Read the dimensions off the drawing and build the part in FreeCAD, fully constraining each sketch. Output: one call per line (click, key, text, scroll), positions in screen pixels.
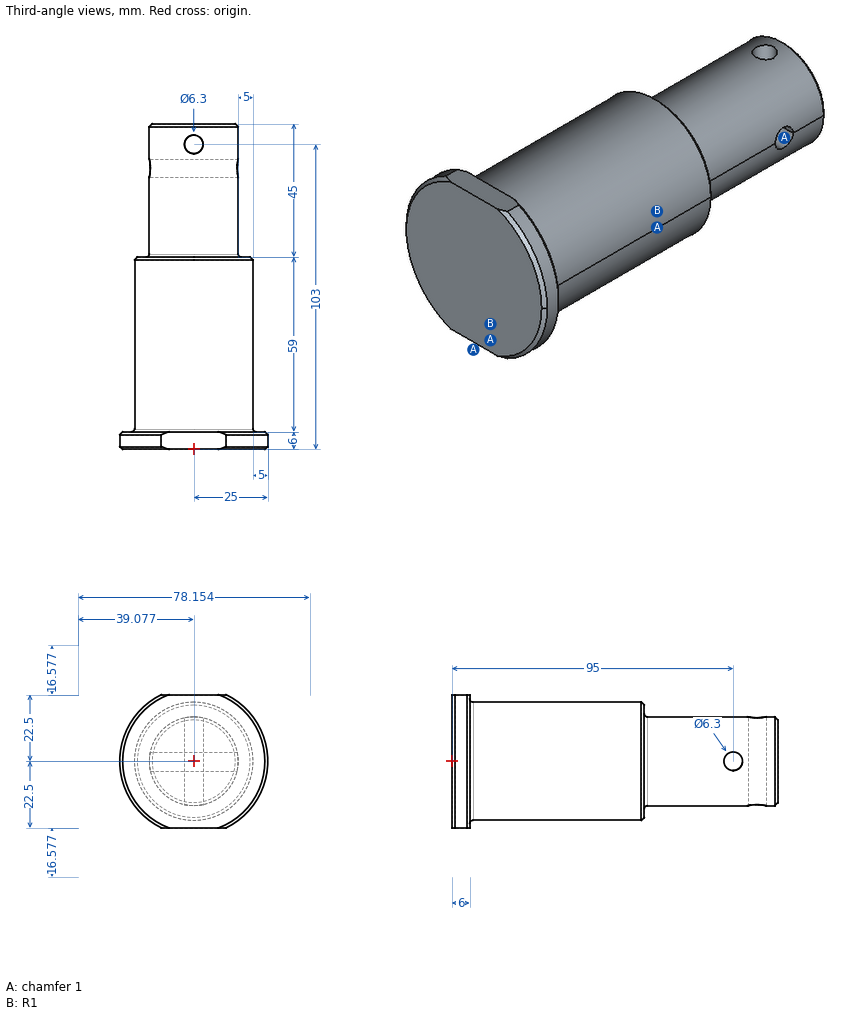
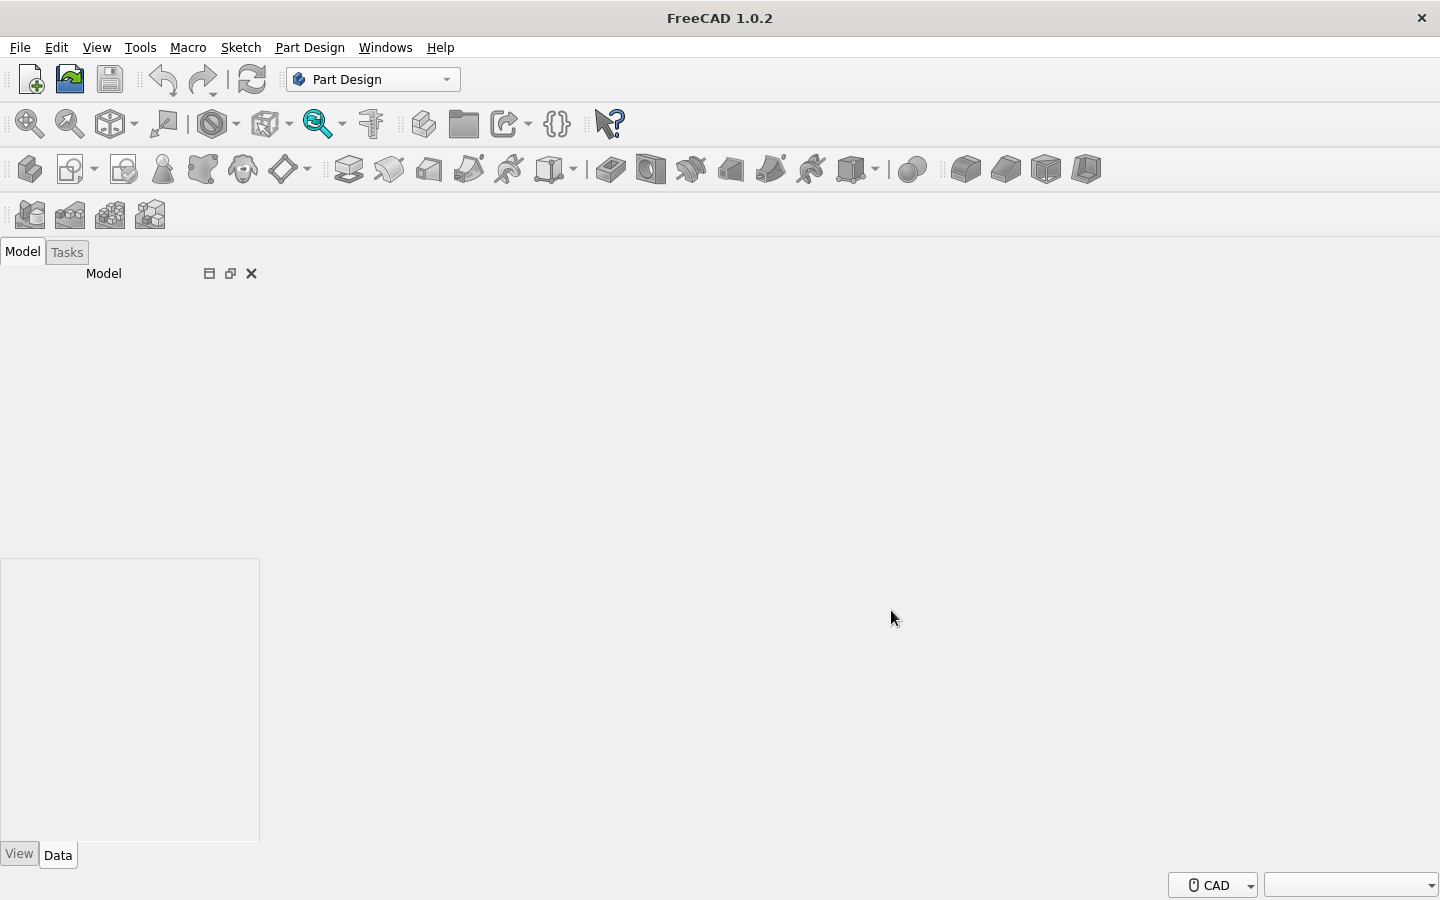
key(ctrl+n)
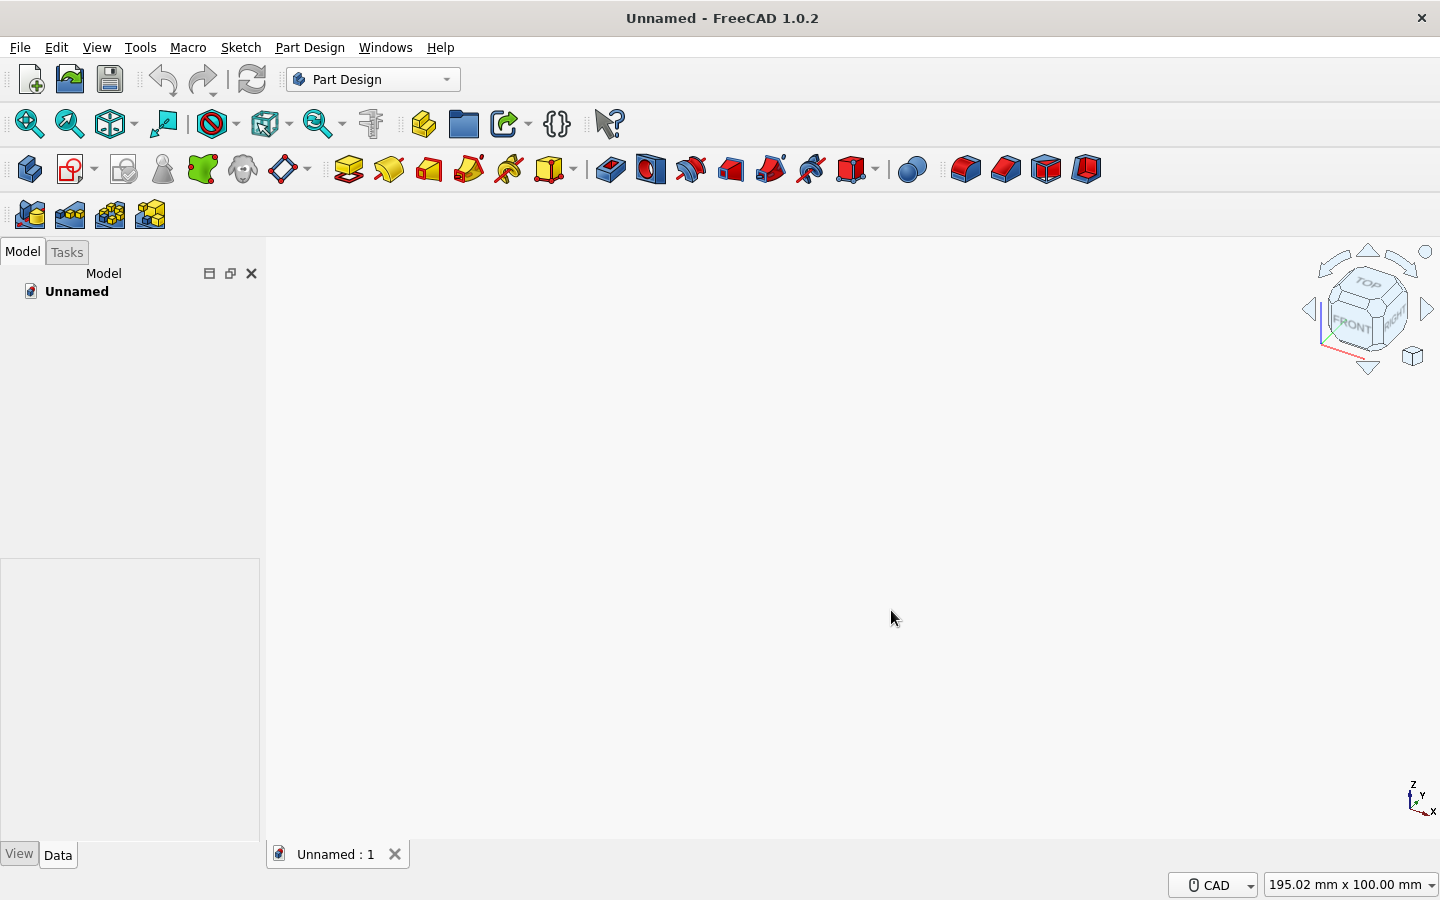
click(70, 170)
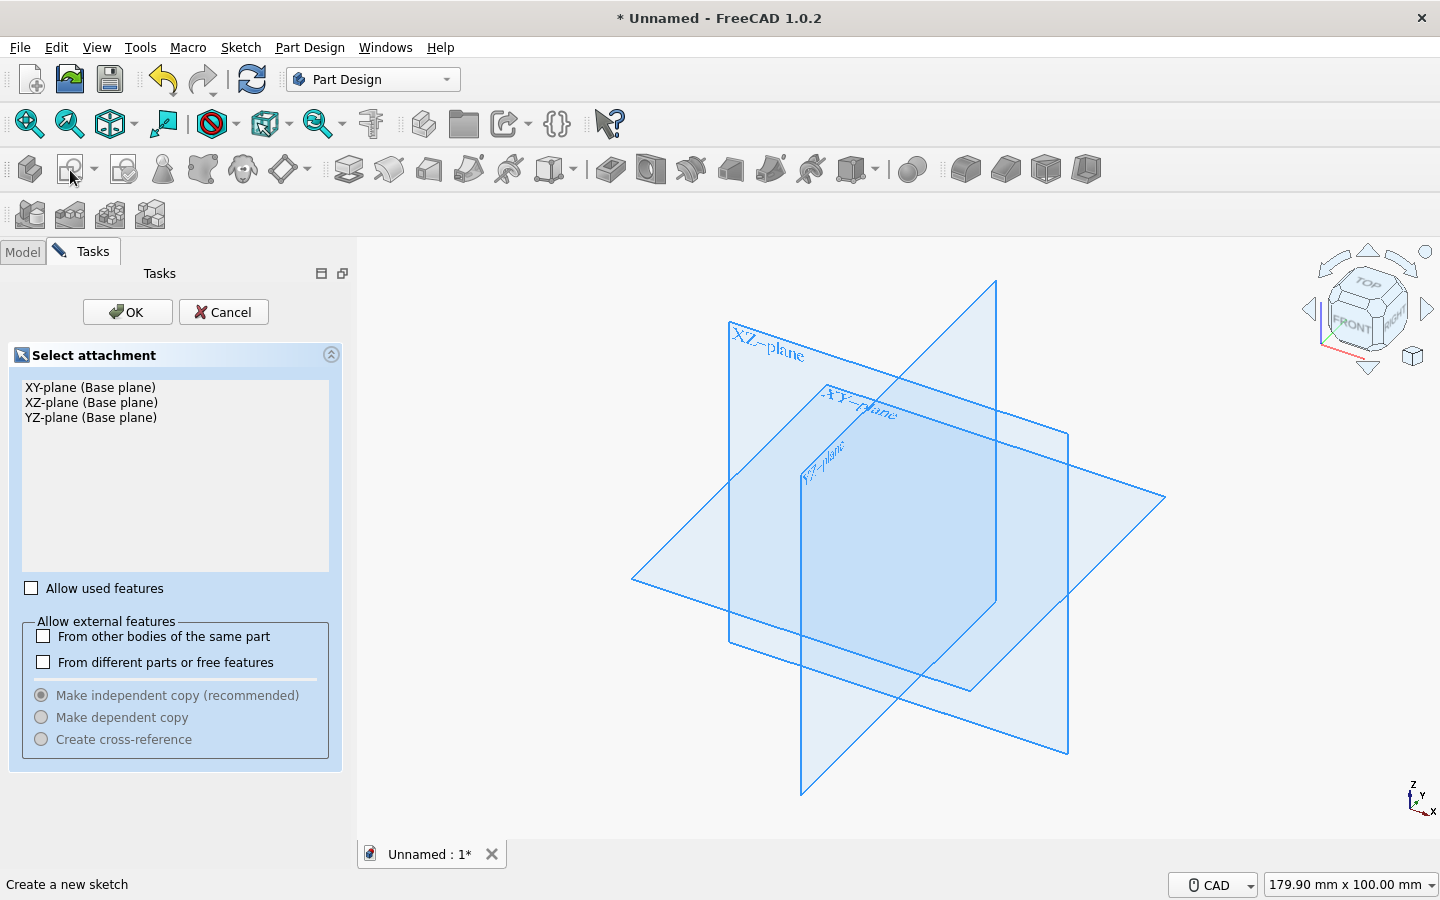
click(82, 388)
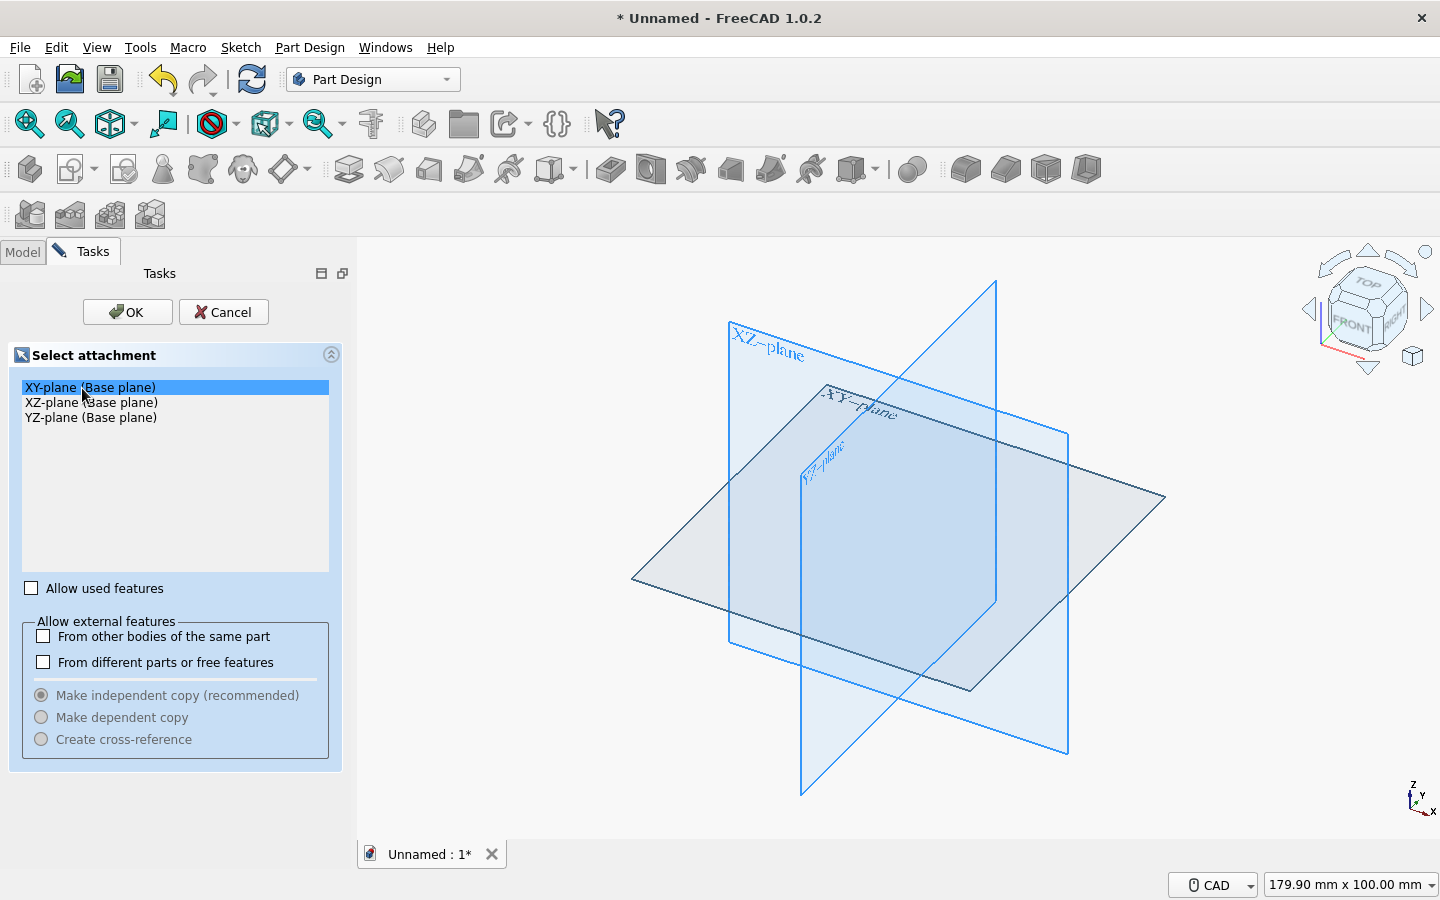
click(128, 312)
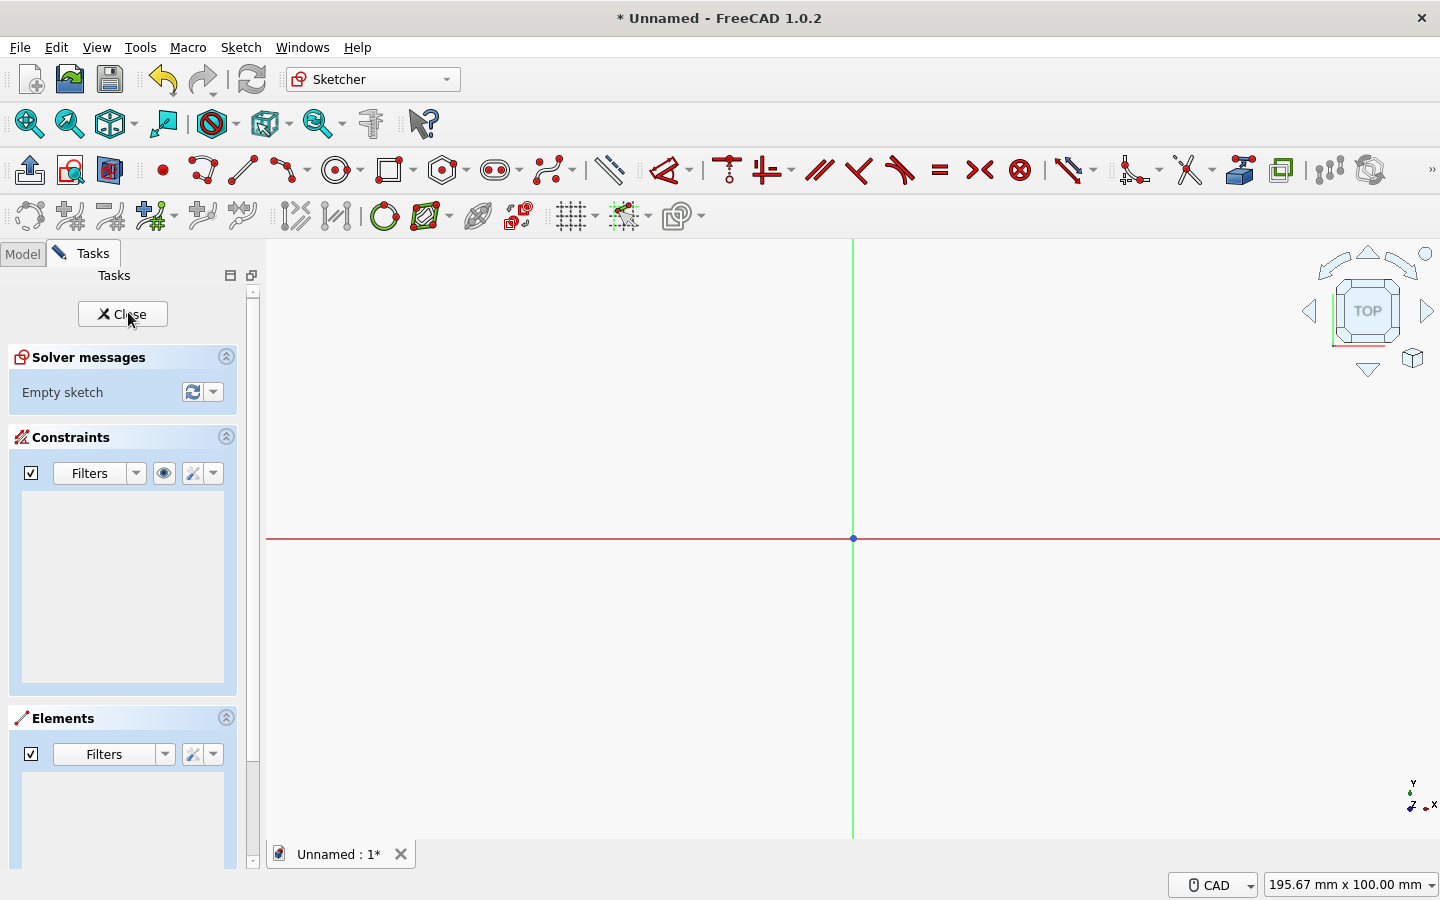
scroll(610, 811, down, 3)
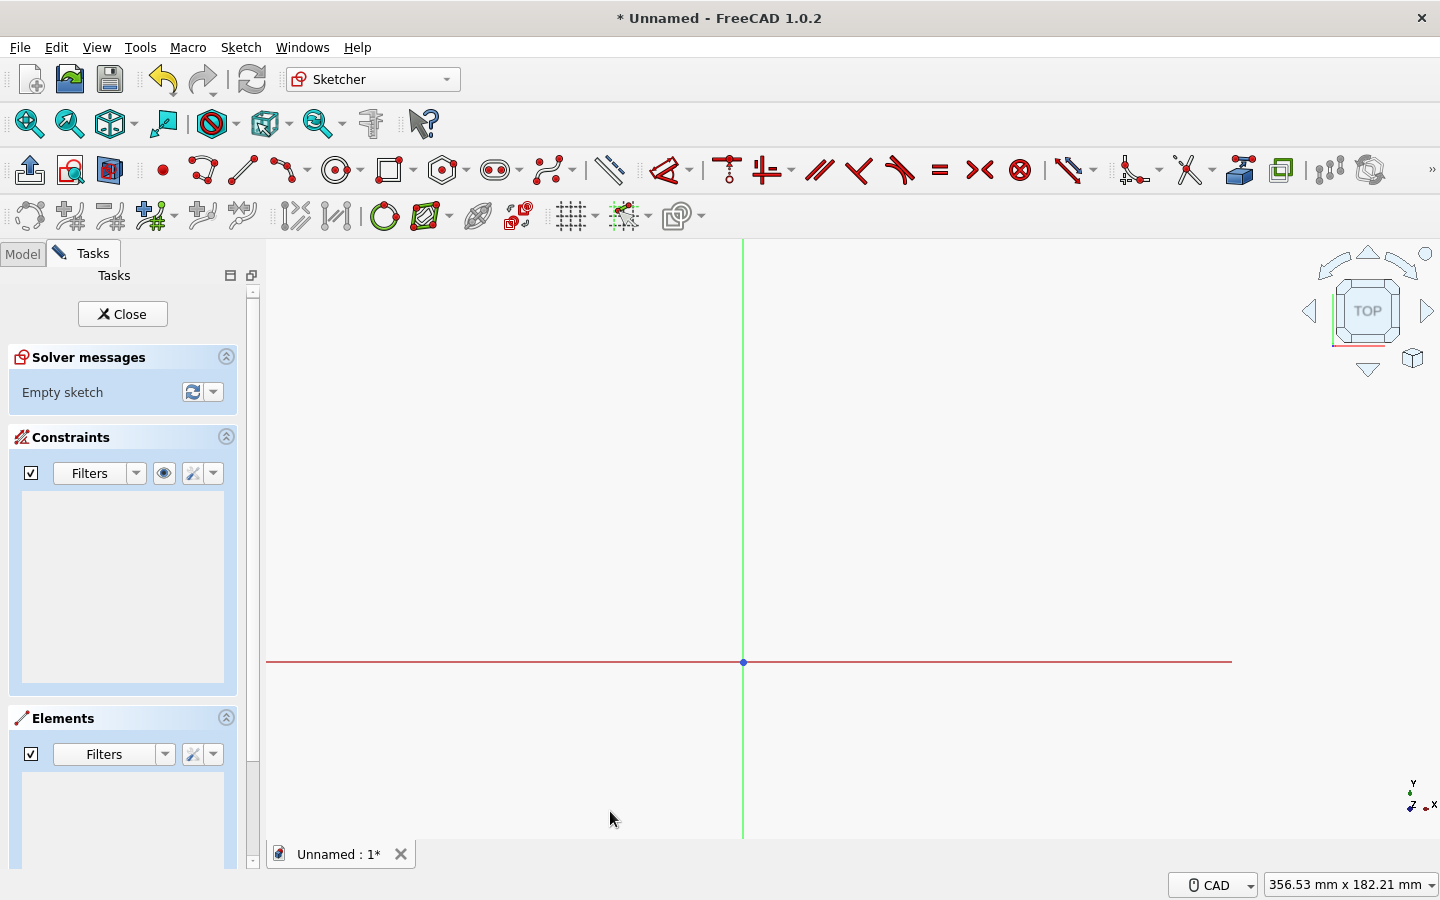
click(204, 170)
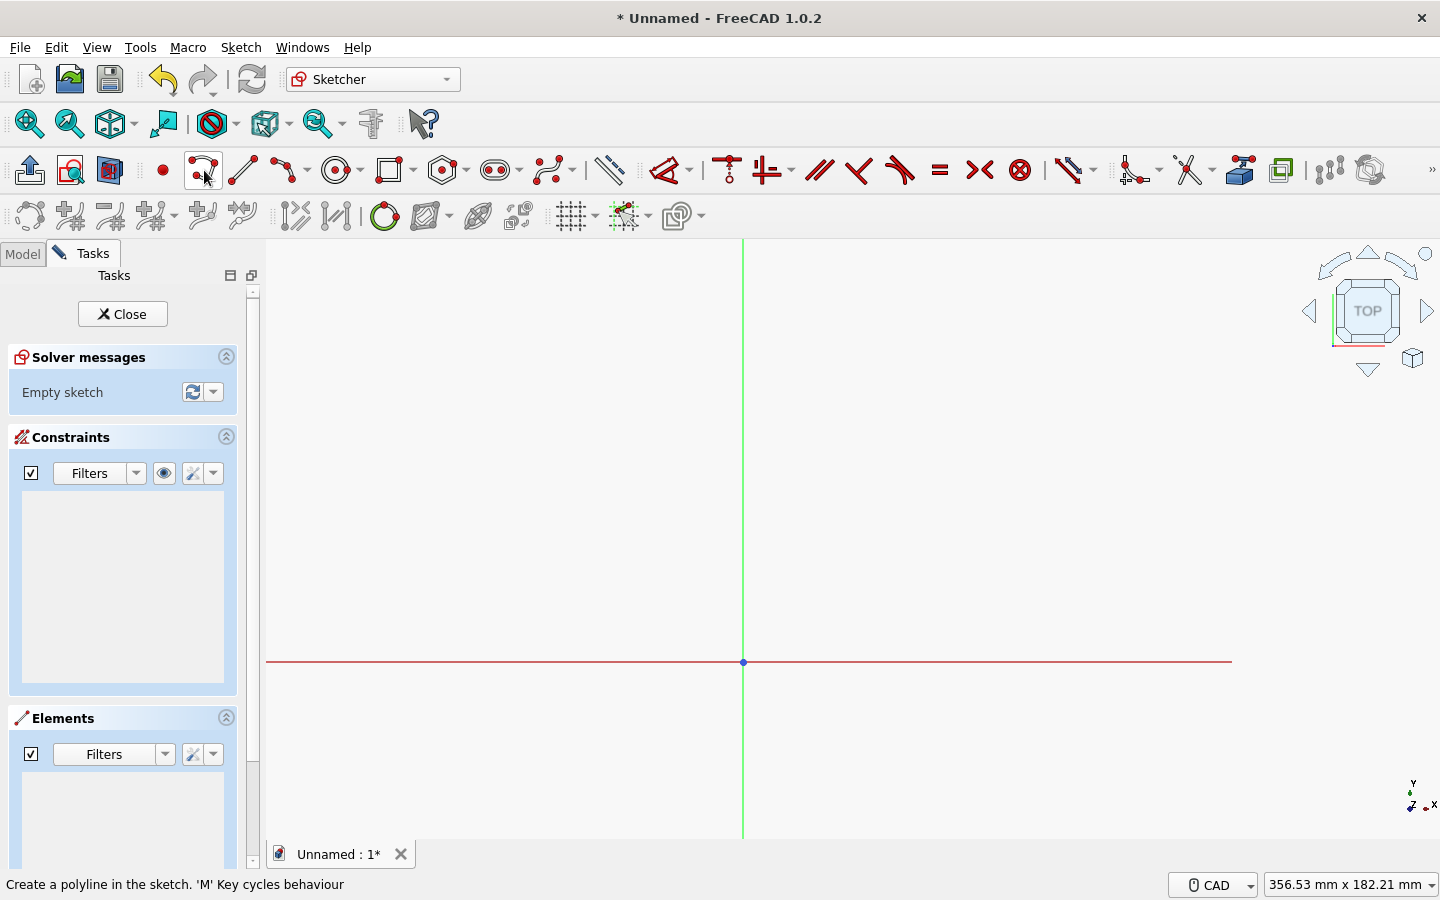
click(743, 662)
click(826, 653)
click(826, 642)
click(809, 642)
click(809, 448)
click(793, 448)
click(793, 300)
click(752, 300)
click(743, 662)
key(Escape)
key(Escape)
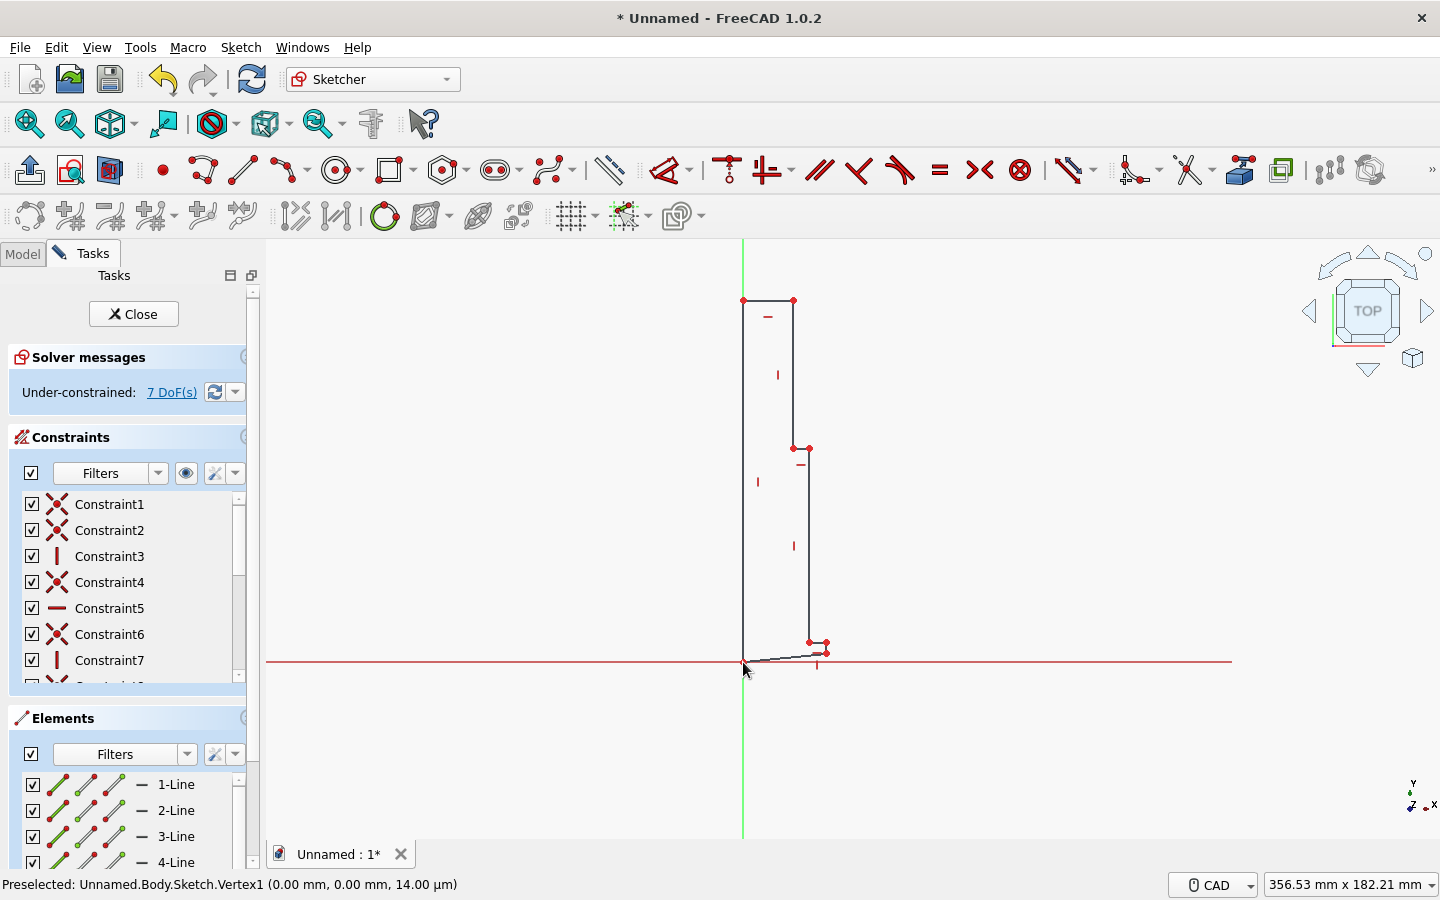
click(768, 660)